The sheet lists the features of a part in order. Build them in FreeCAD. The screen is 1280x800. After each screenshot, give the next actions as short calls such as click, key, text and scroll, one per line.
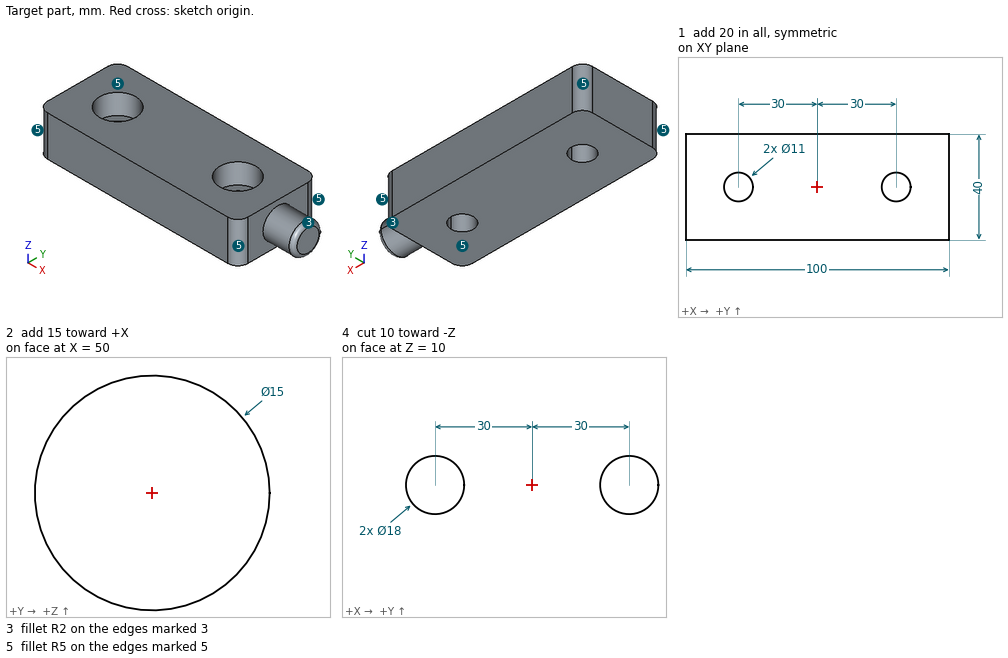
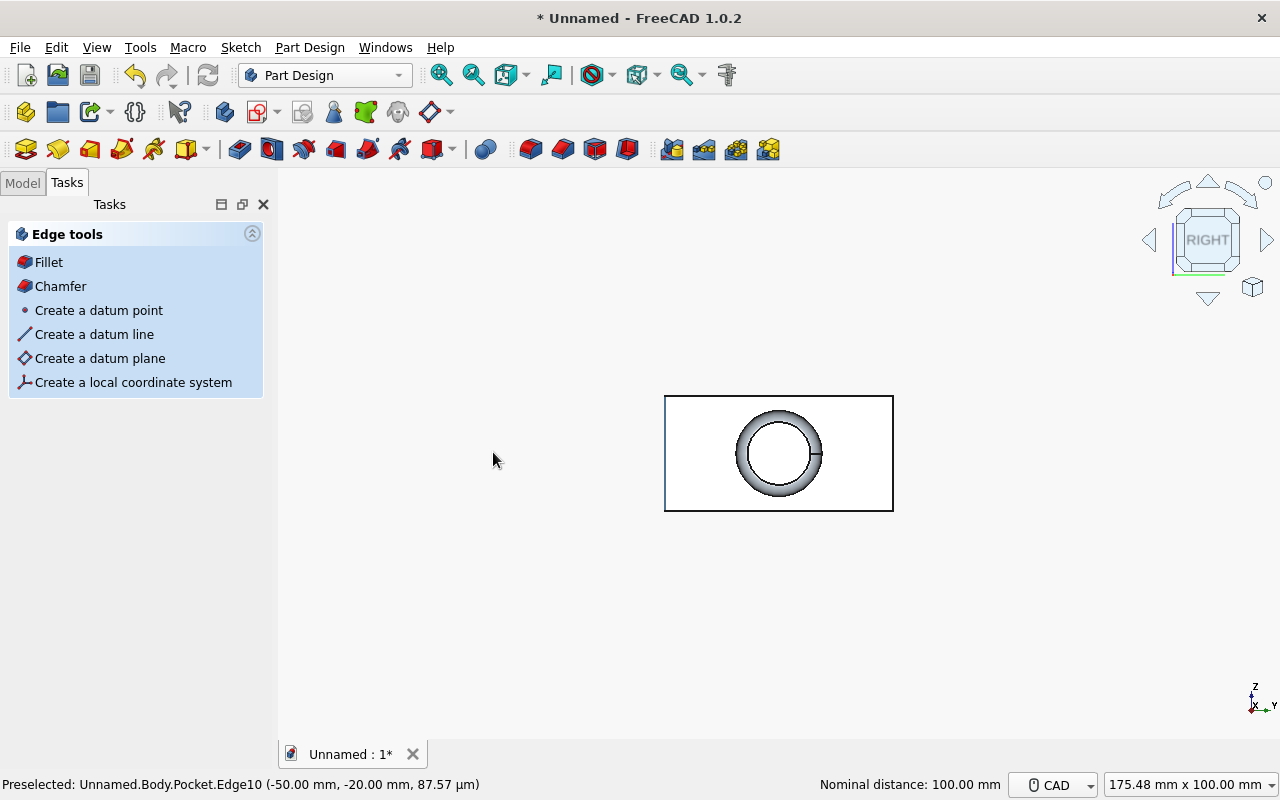
key(v)
key(f)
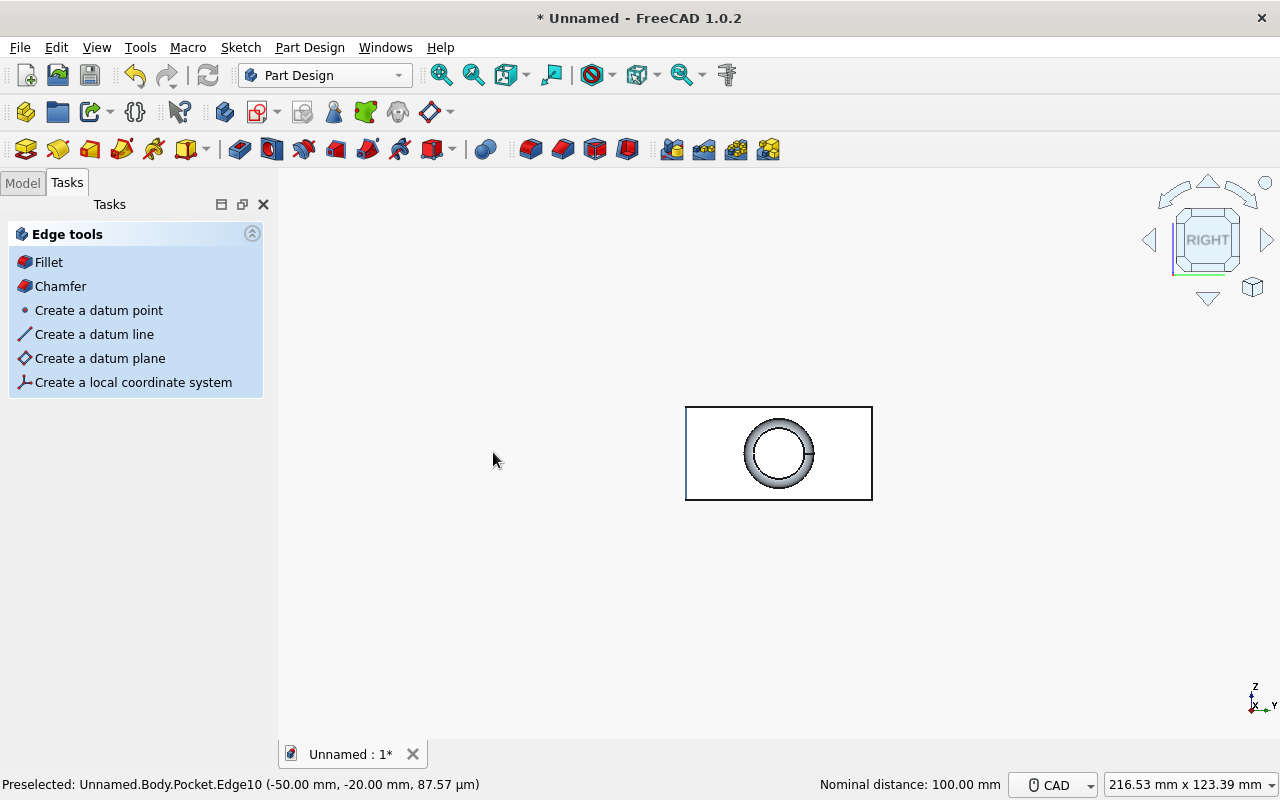
click(872, 452, ctrl)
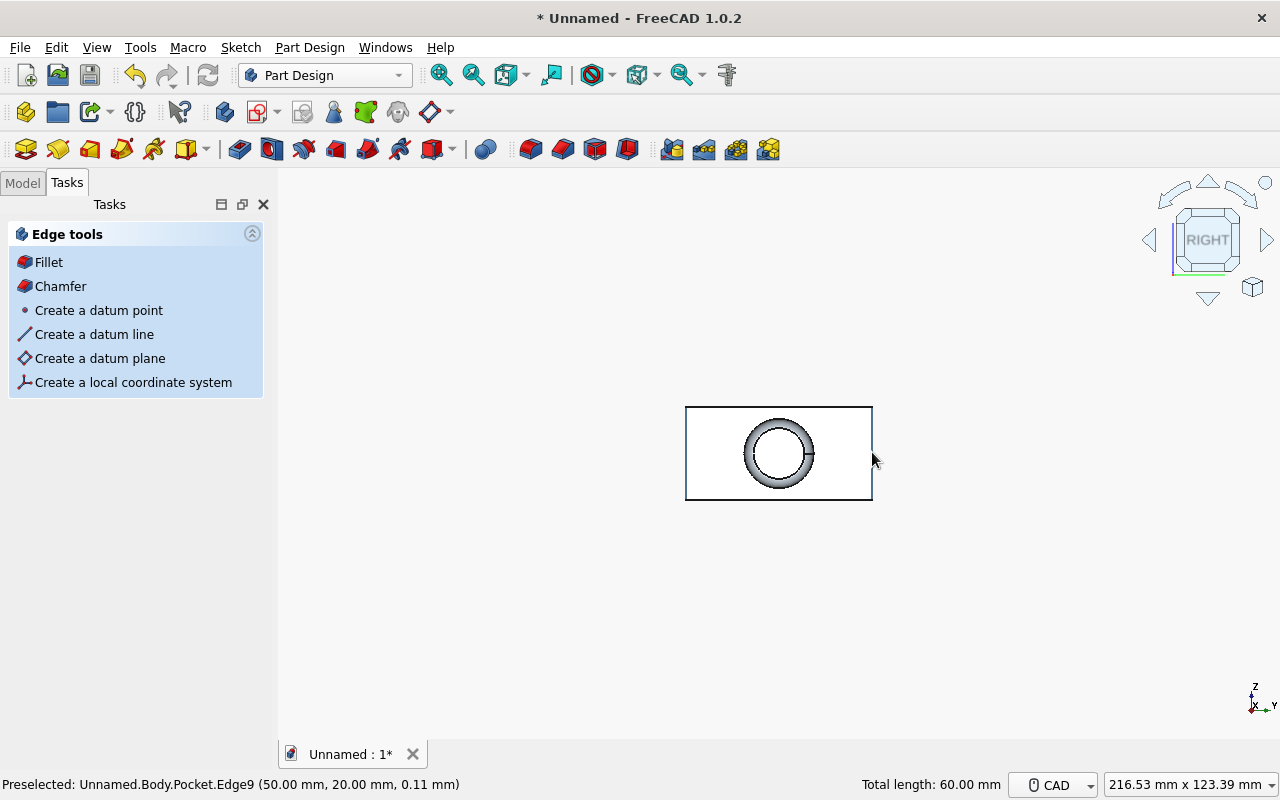
key(5)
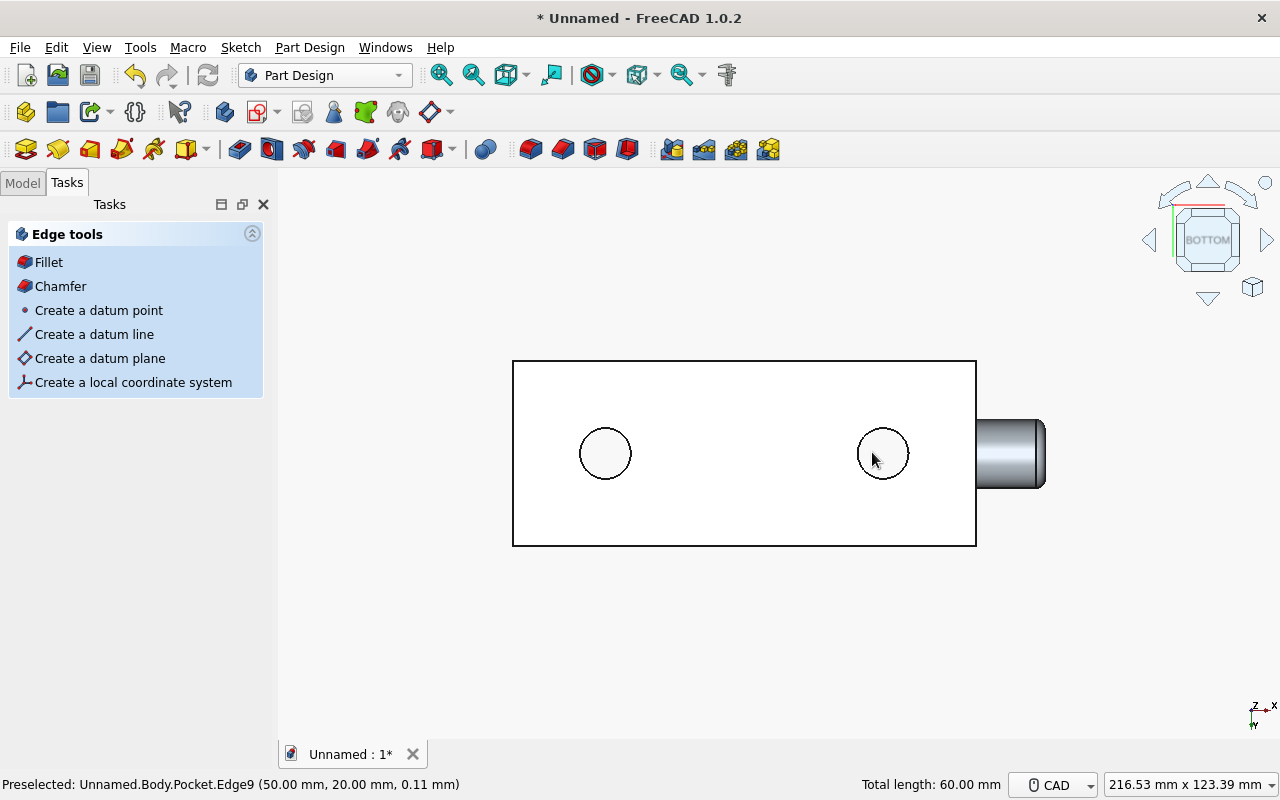
key(4)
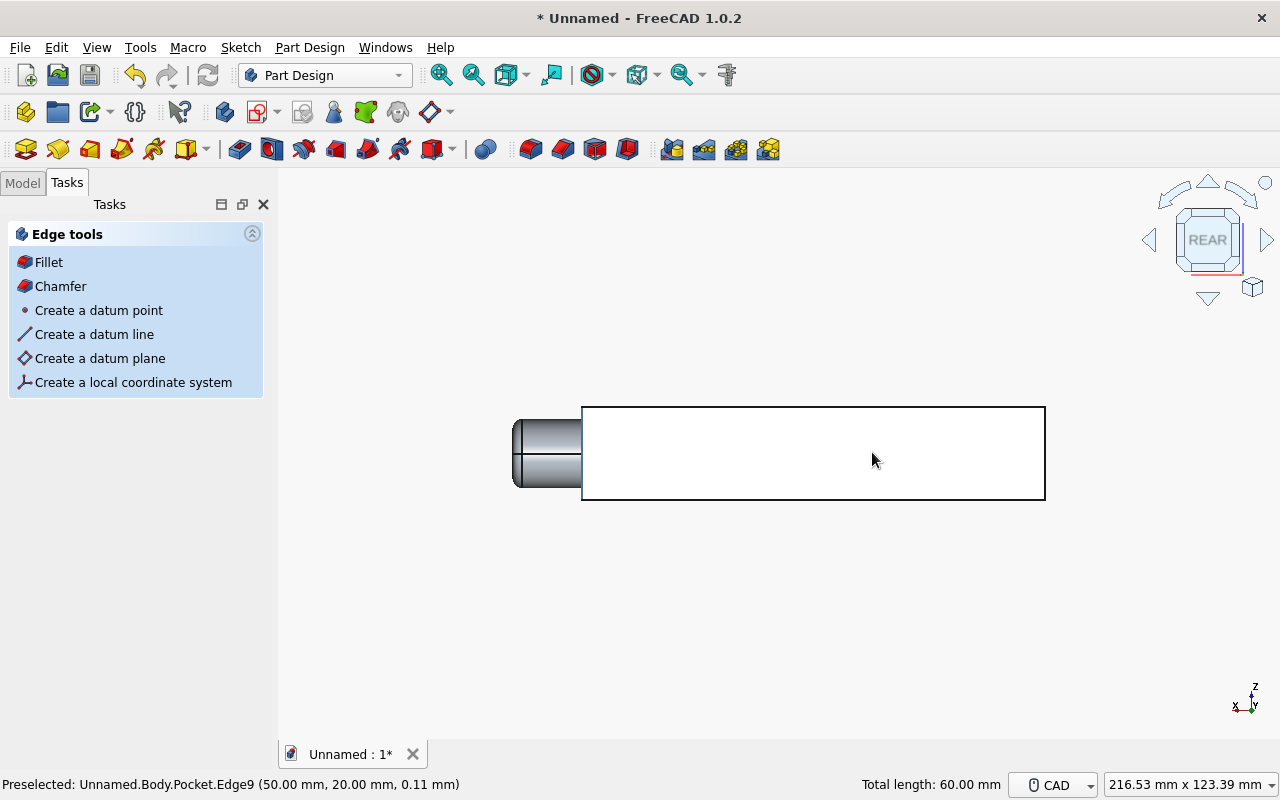
click(1045, 452, ctrl)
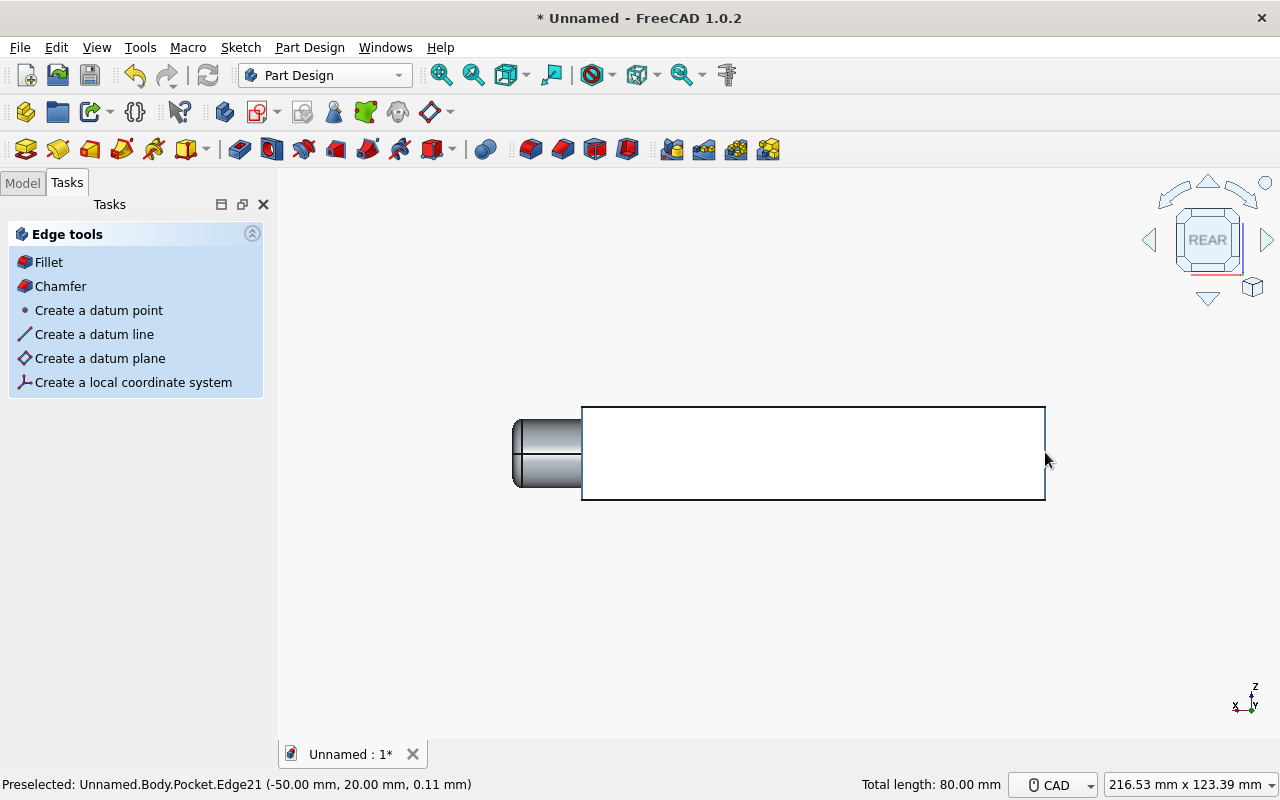
click(532, 150)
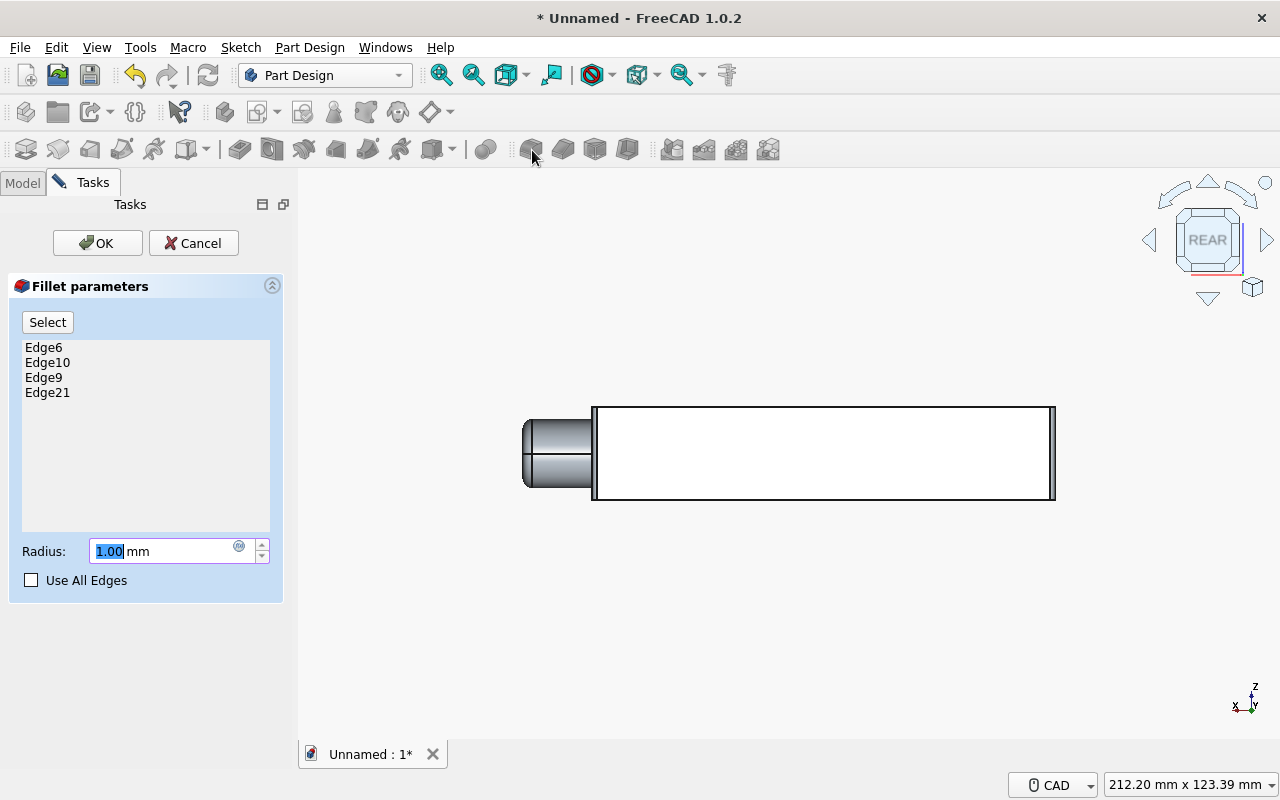
text(5)
key(Tab)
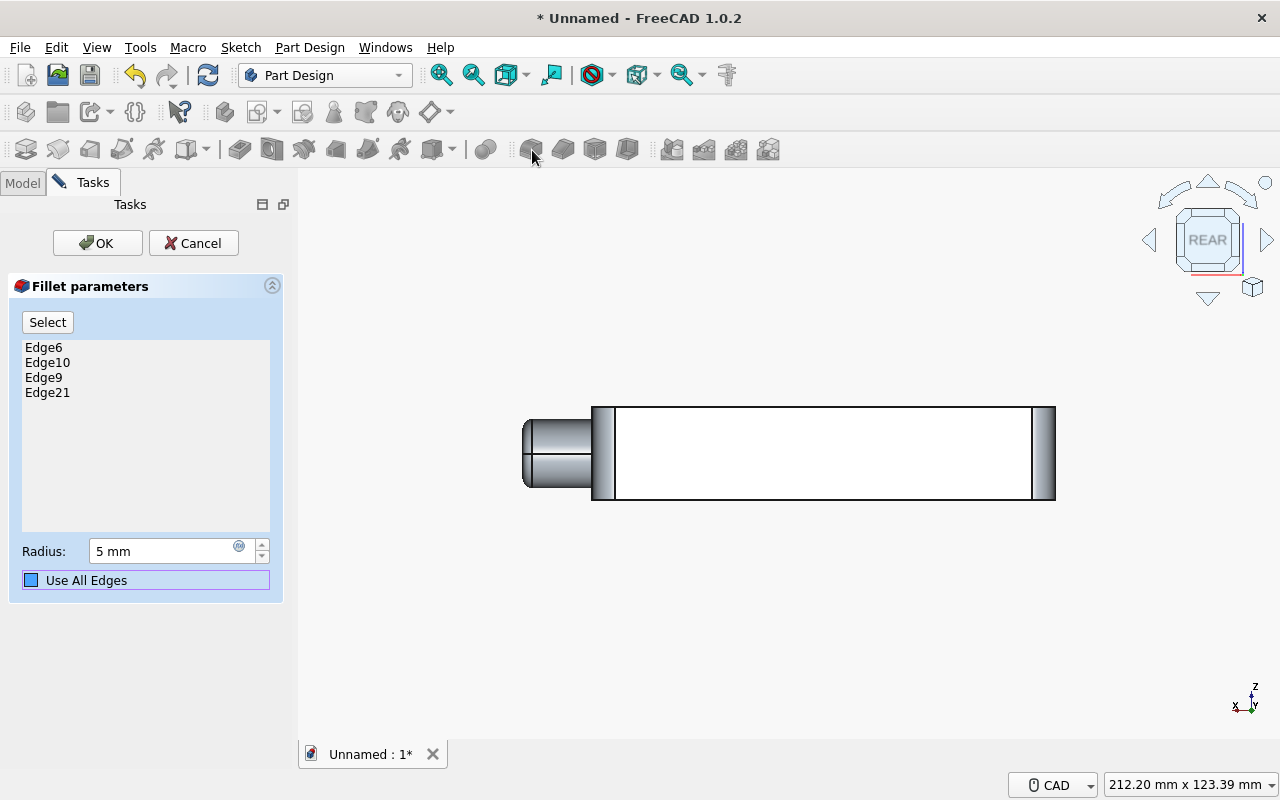
click(98, 243)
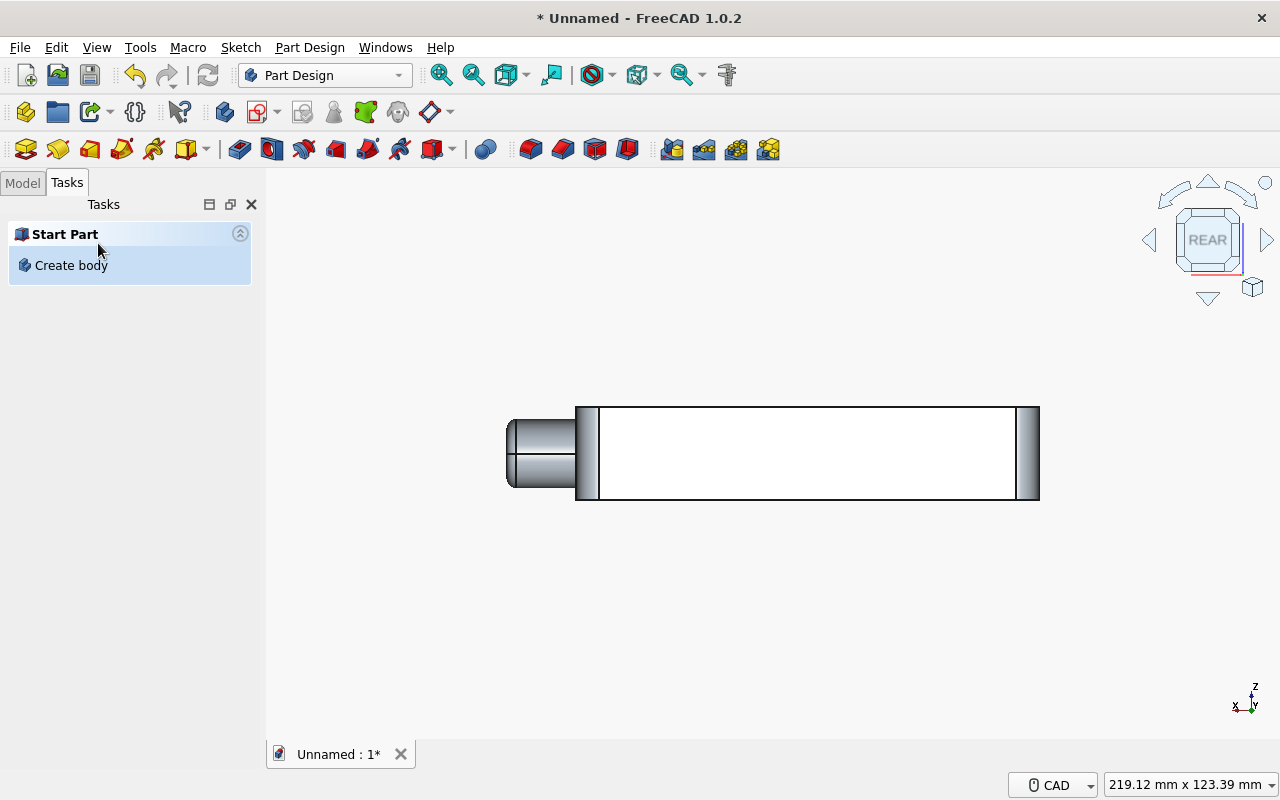
key(0)